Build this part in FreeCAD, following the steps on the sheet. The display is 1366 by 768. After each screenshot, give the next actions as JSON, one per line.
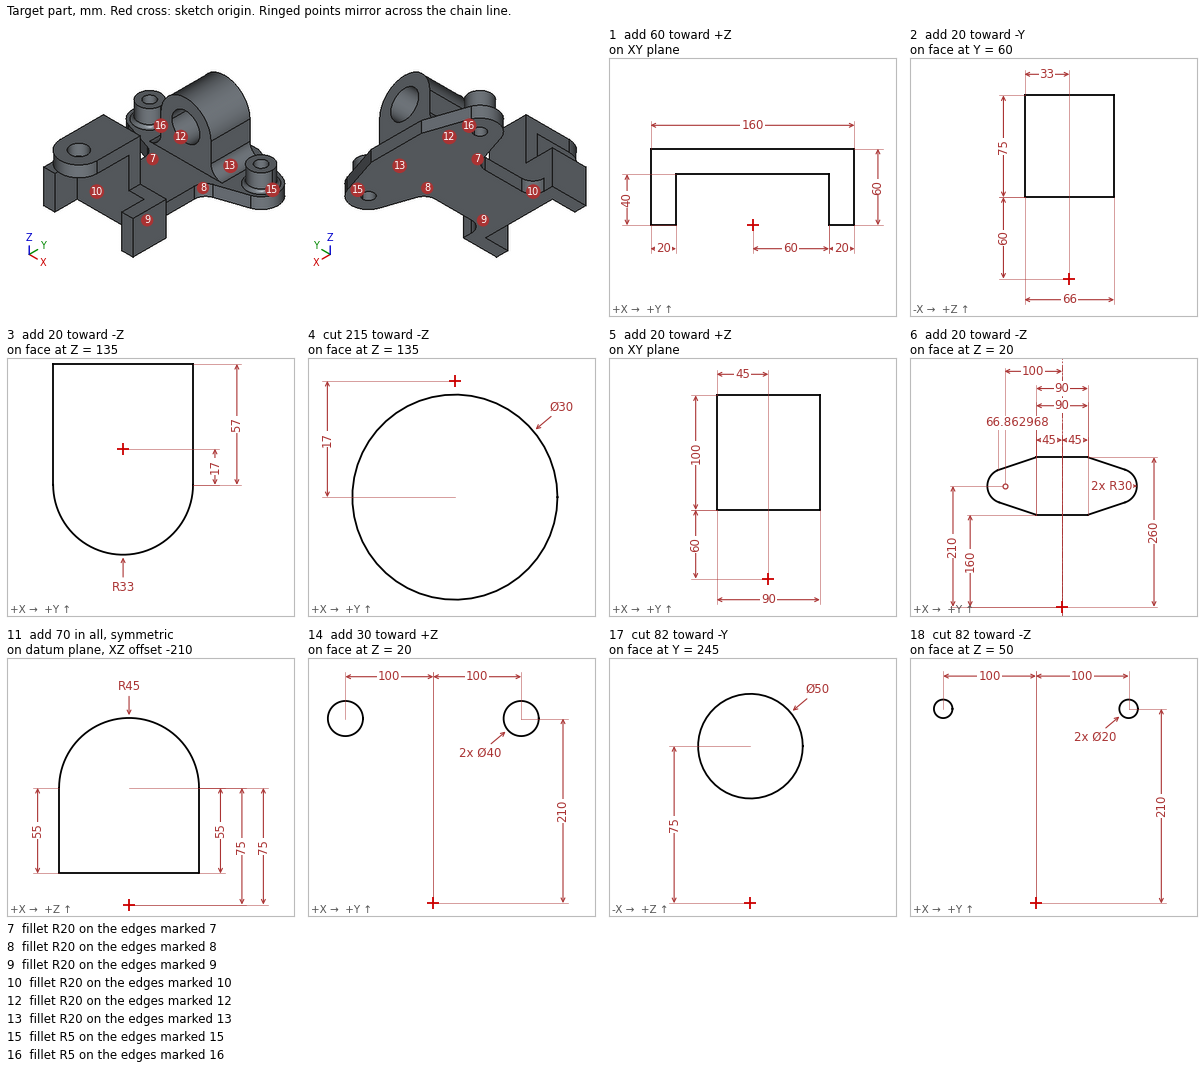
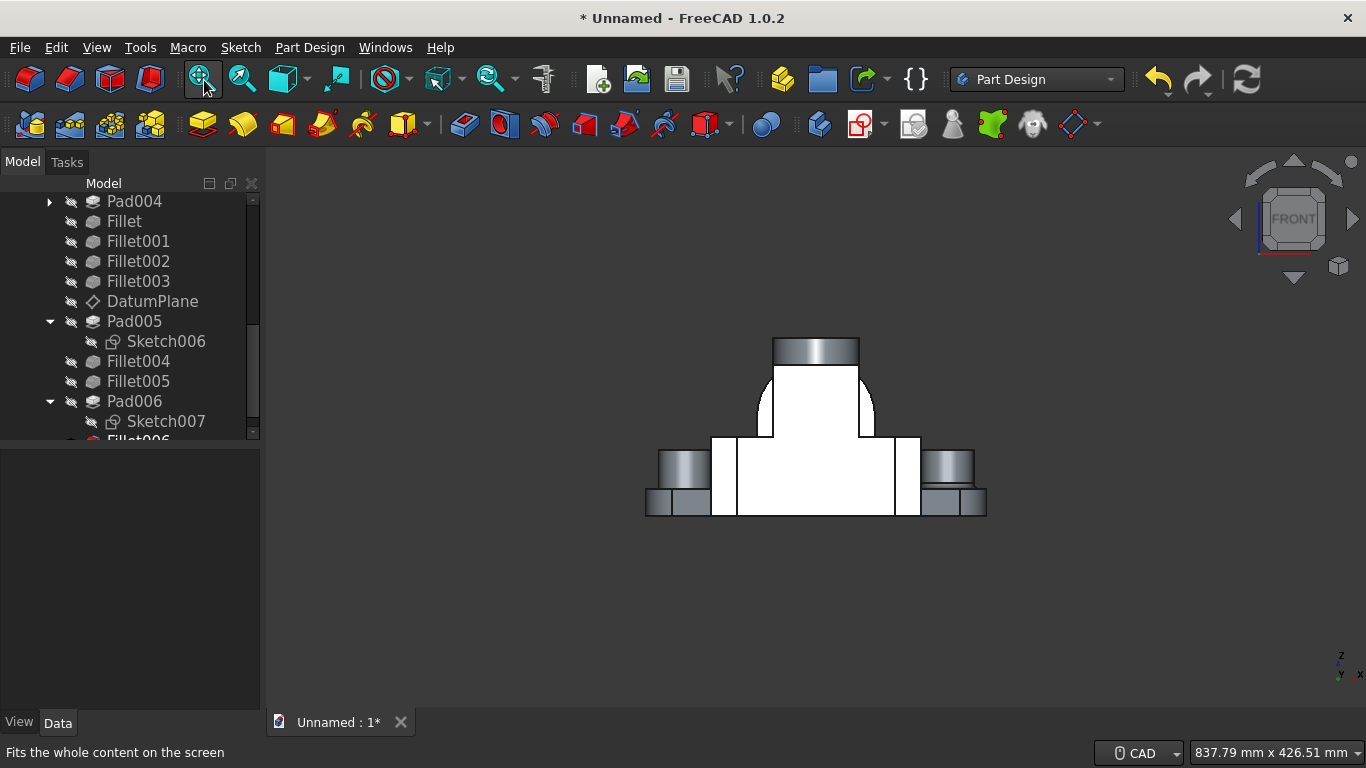
{"action": "key", "text": "3"}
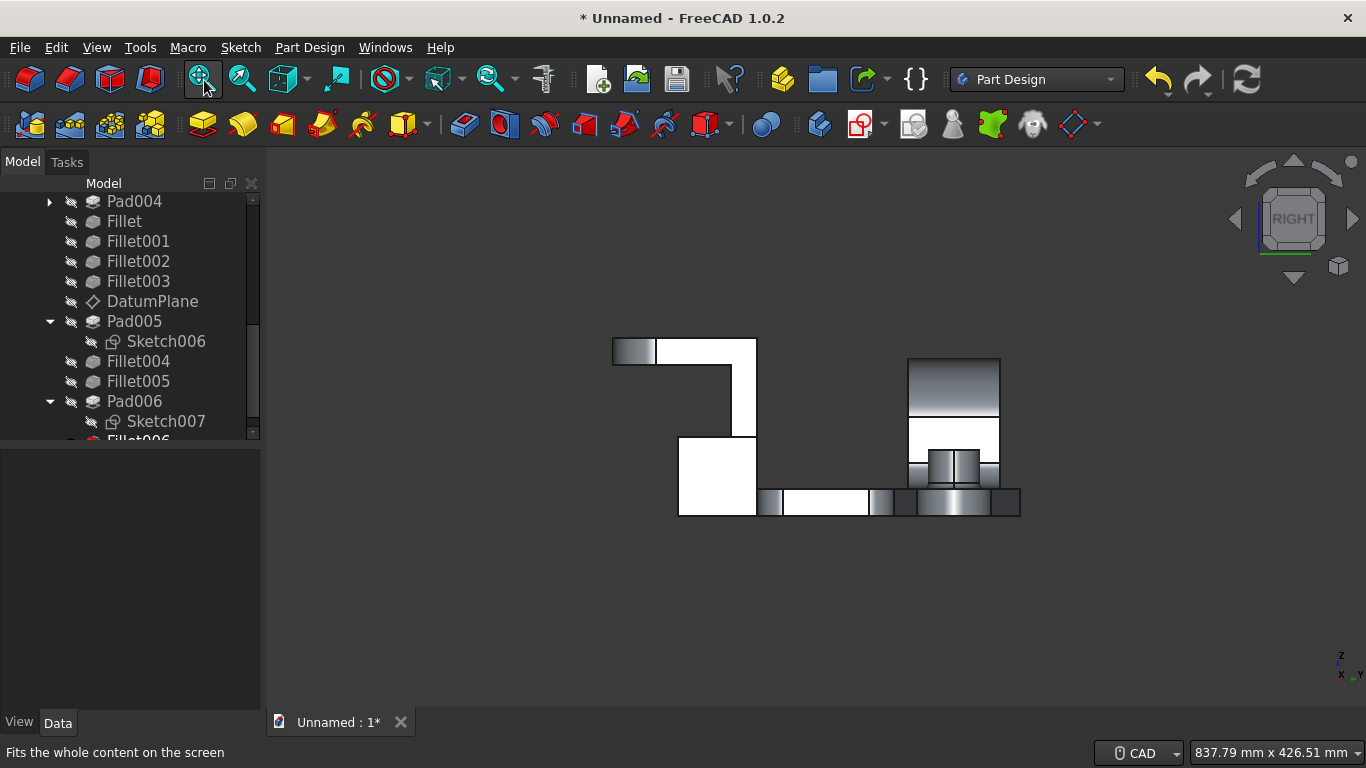
{"action": "left_click", "coordinate": [204, 80]}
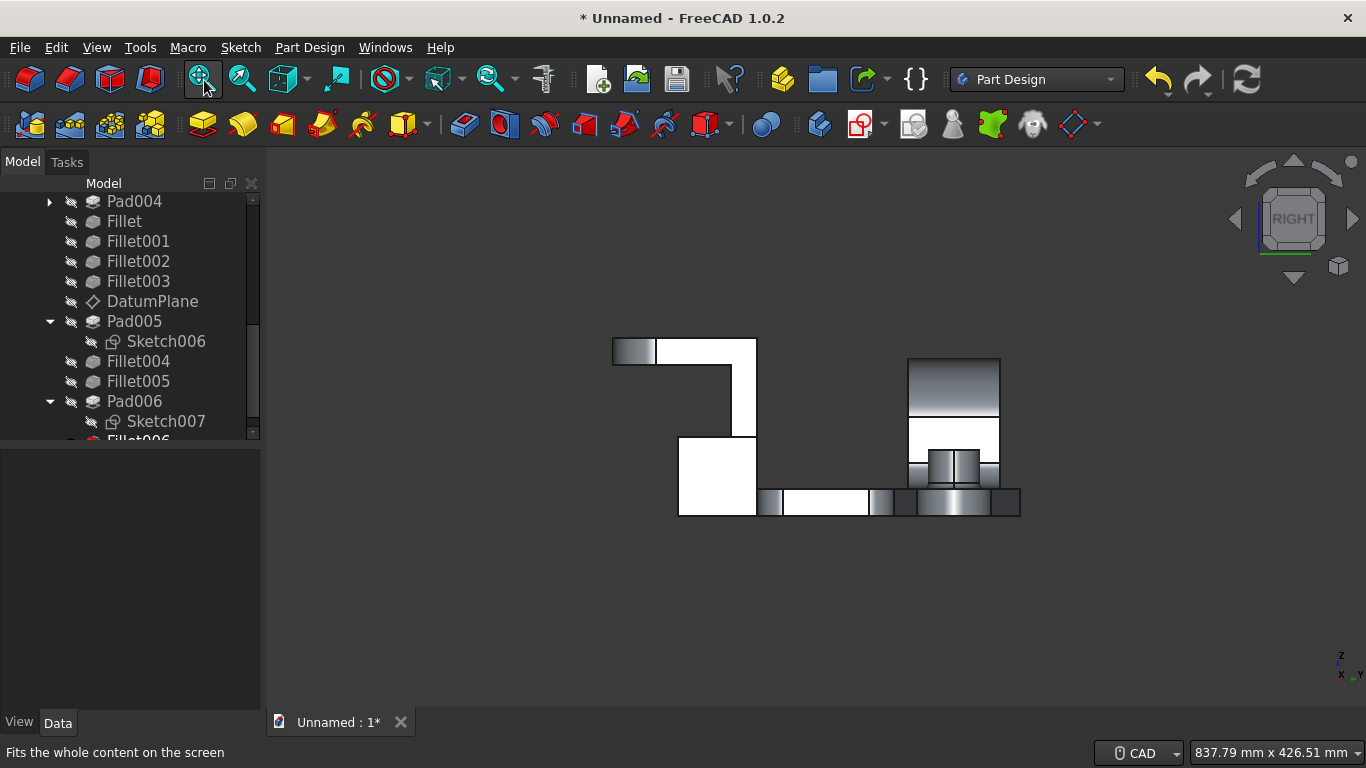
{"action": "key", "text": "5"}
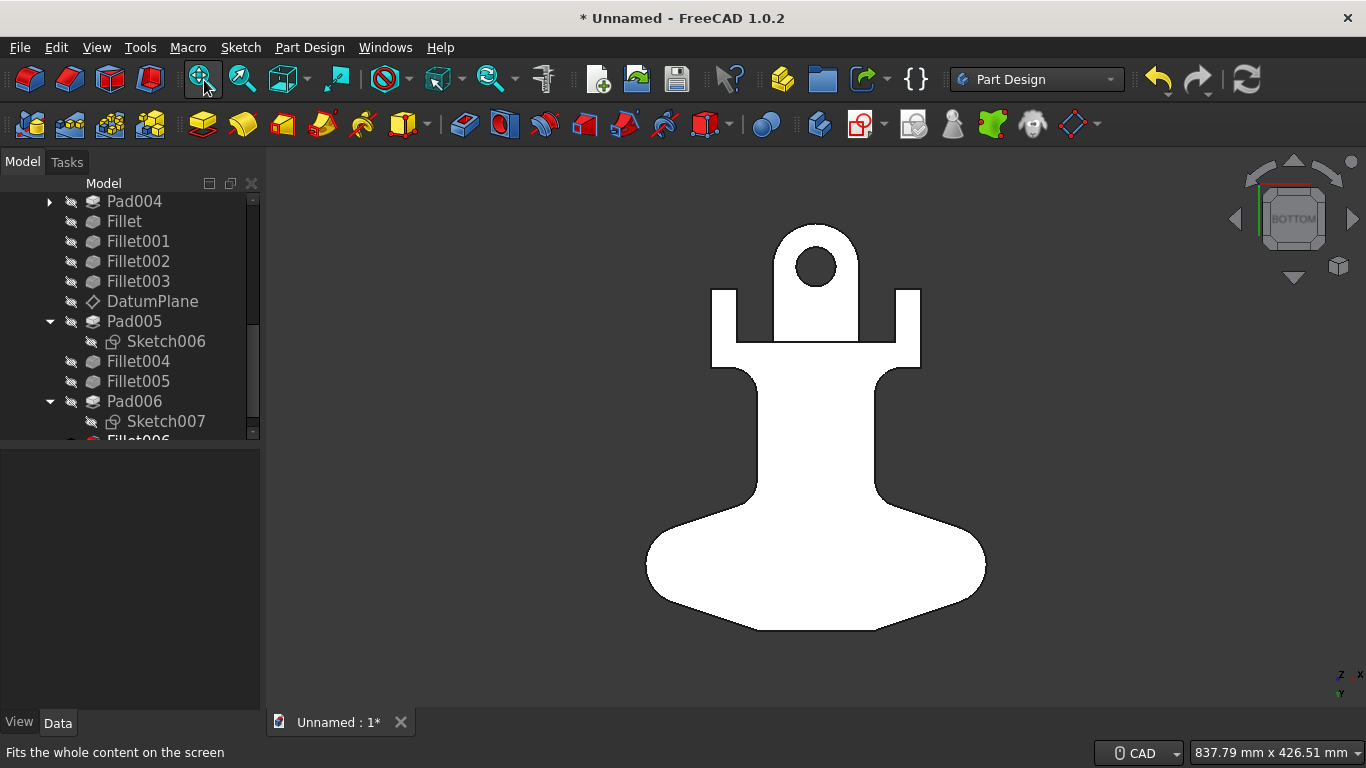
{"action": "key", "text": "4"}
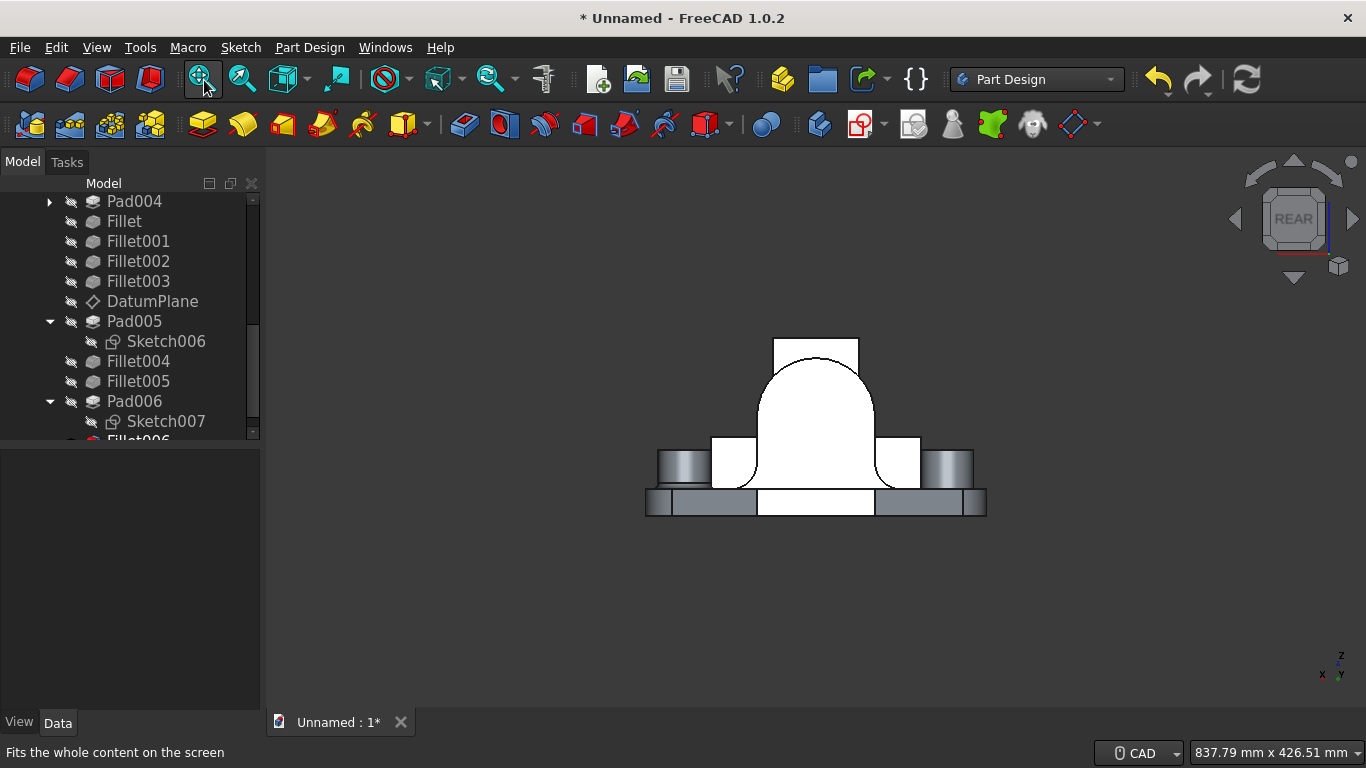
{"action": "left_click", "coordinate": [204, 80]}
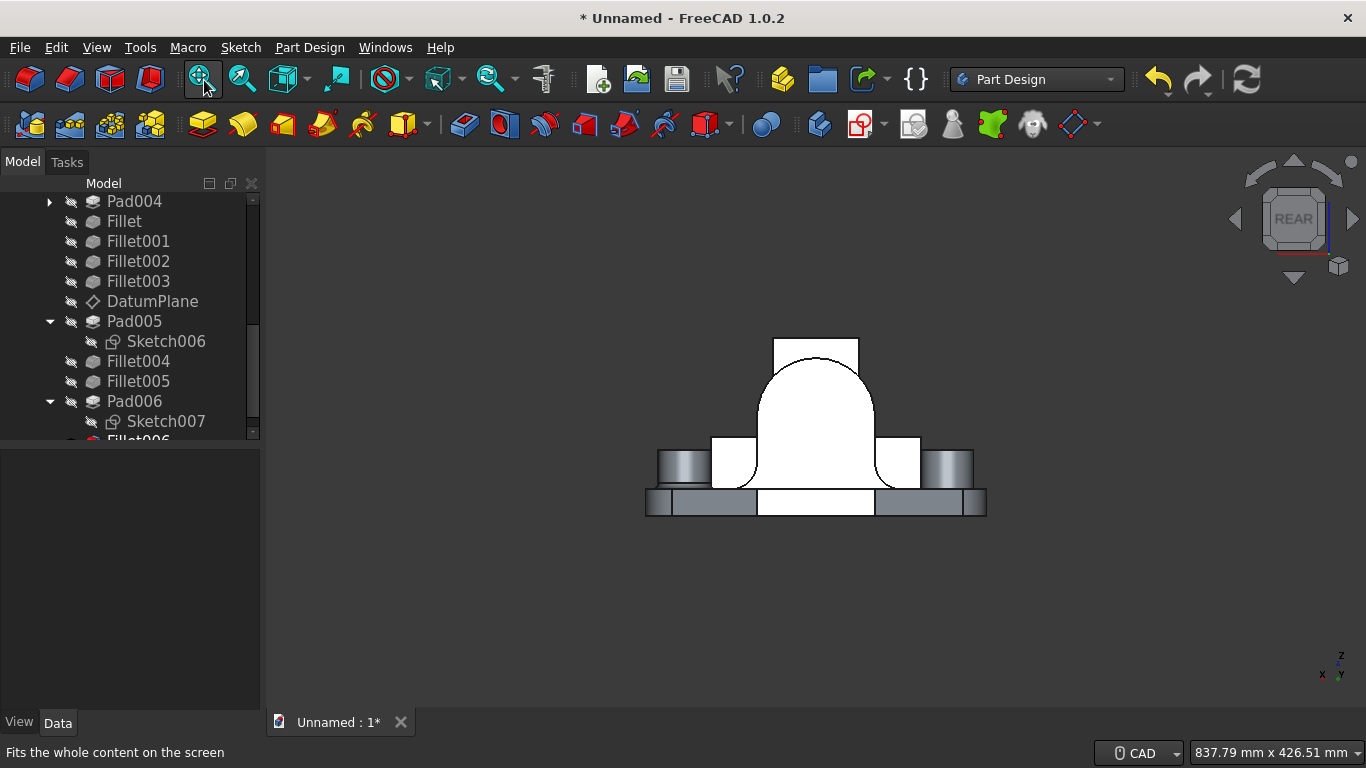
{"action": "key", "text": "6"}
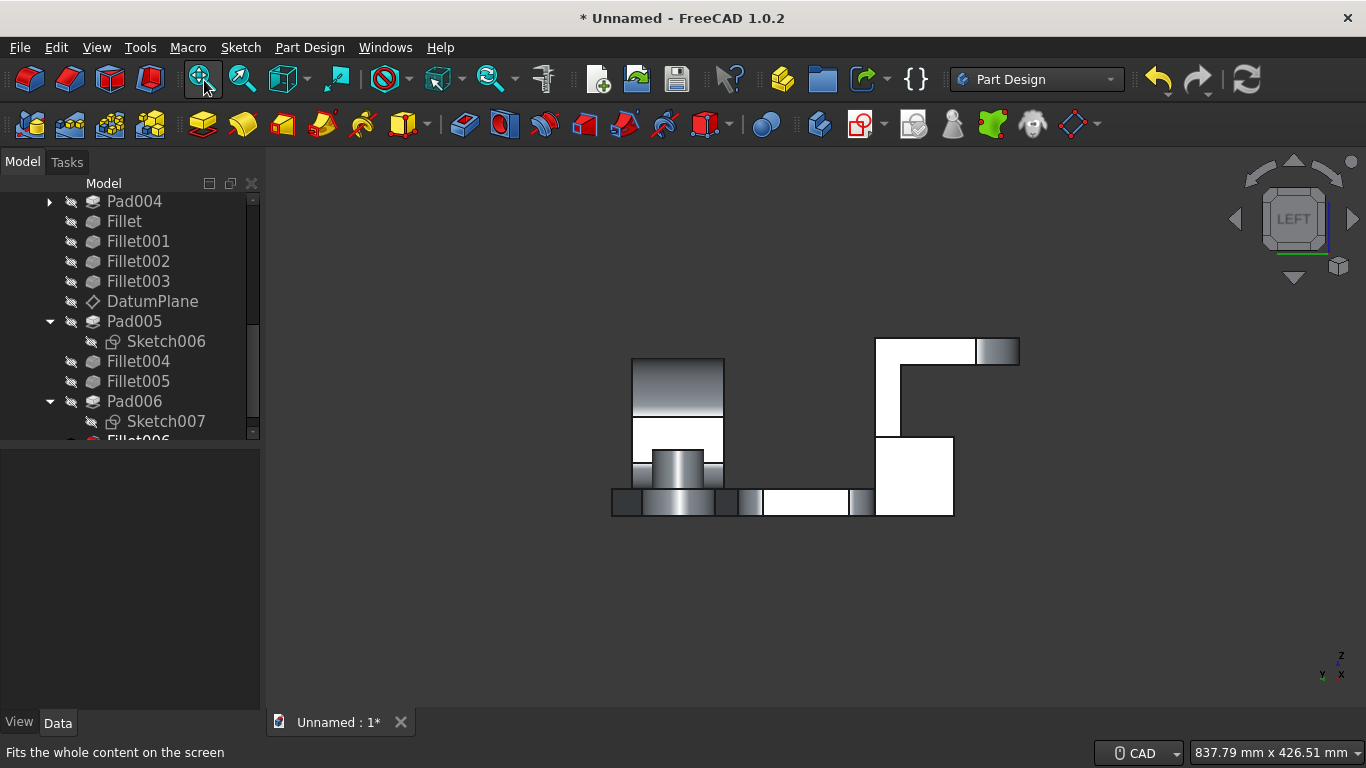
{"action": "key", "text": "v f"}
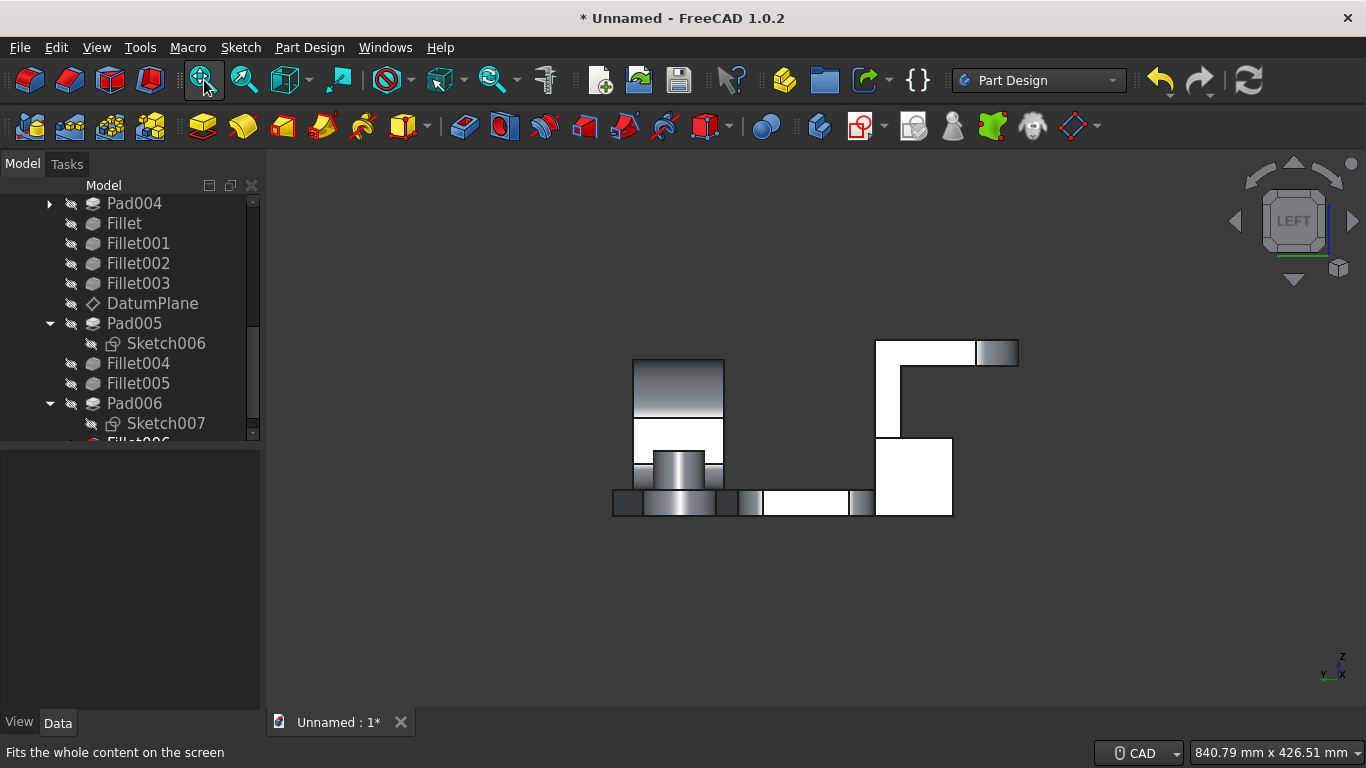
{"action": "key", "text": "v 3"}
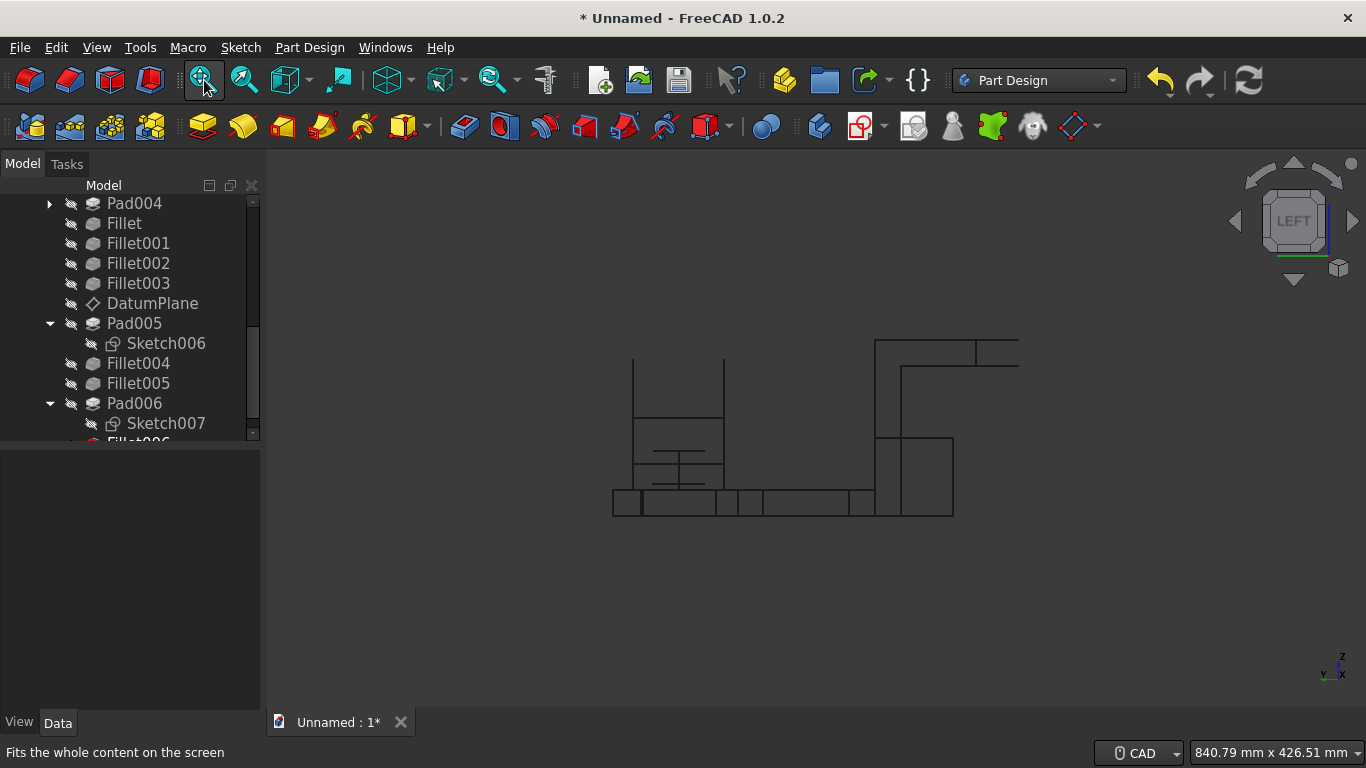
{"action": "key", "text": "0"}